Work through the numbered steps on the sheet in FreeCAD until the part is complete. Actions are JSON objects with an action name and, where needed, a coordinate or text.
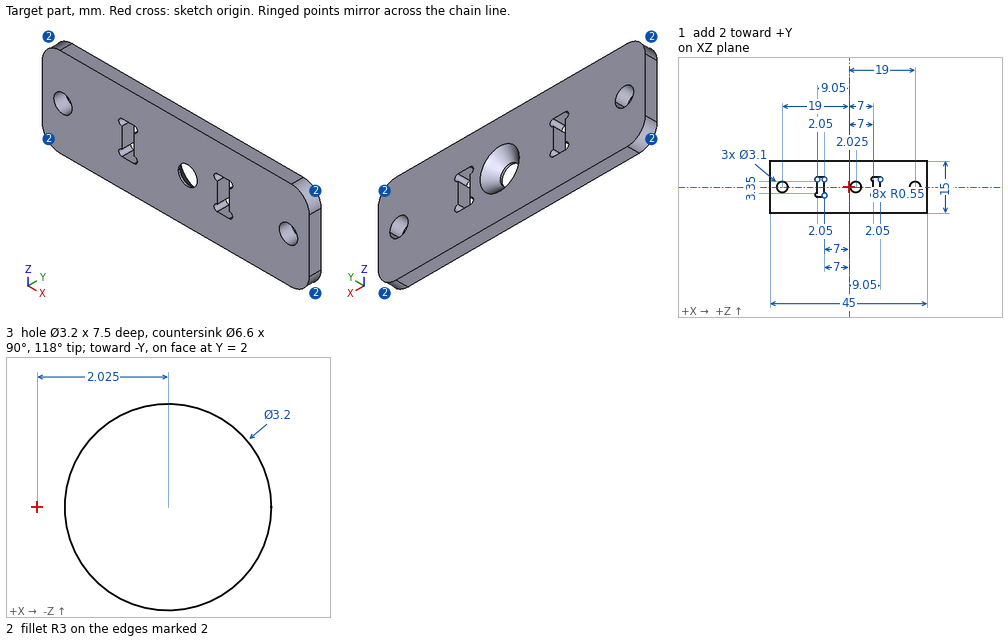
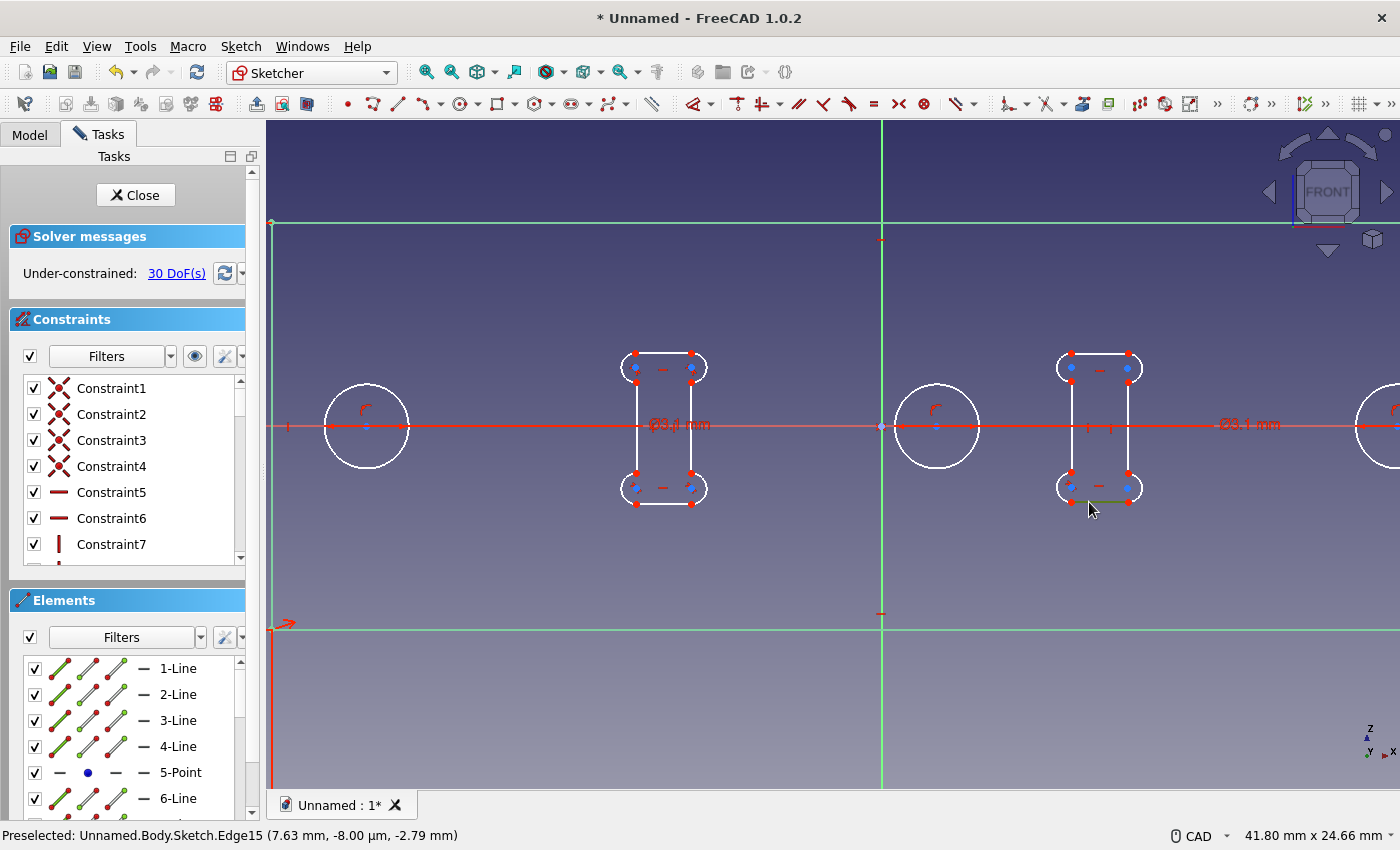
{"action": "left_click", "coordinate": [1139, 496]}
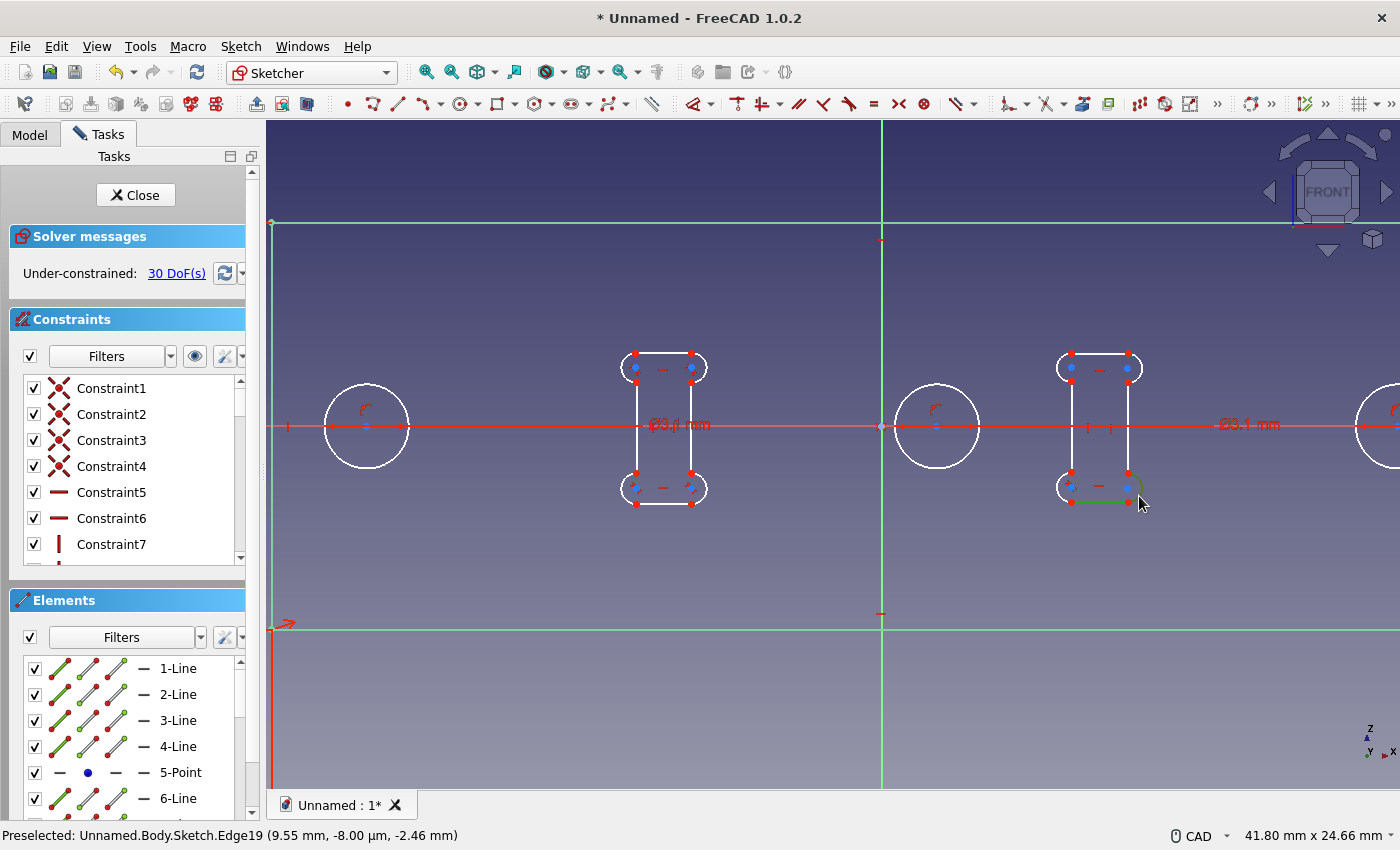
{"action": "left_click", "coordinate": [849, 104]}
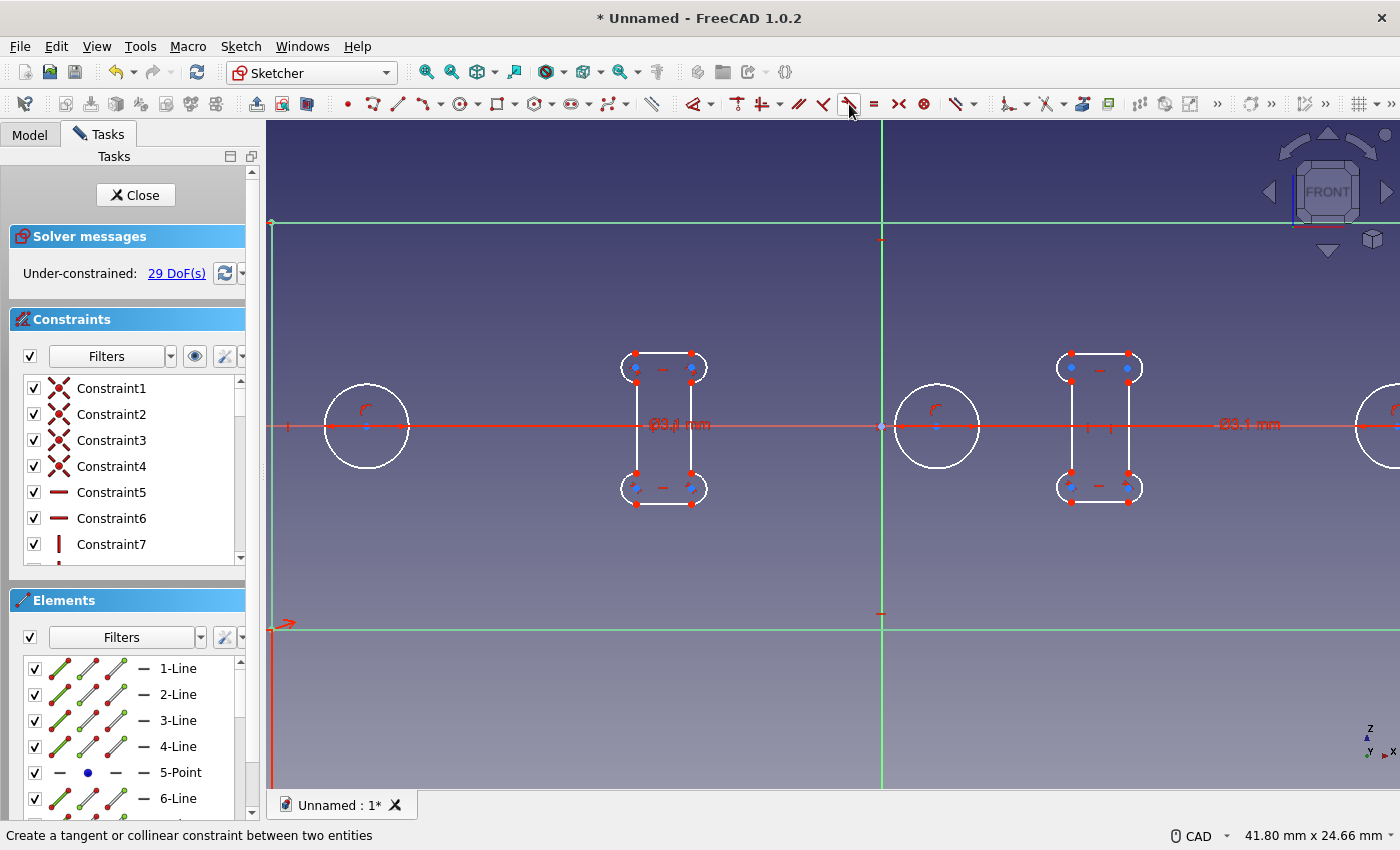
{"action": "left_click", "coordinate": [1112, 354]}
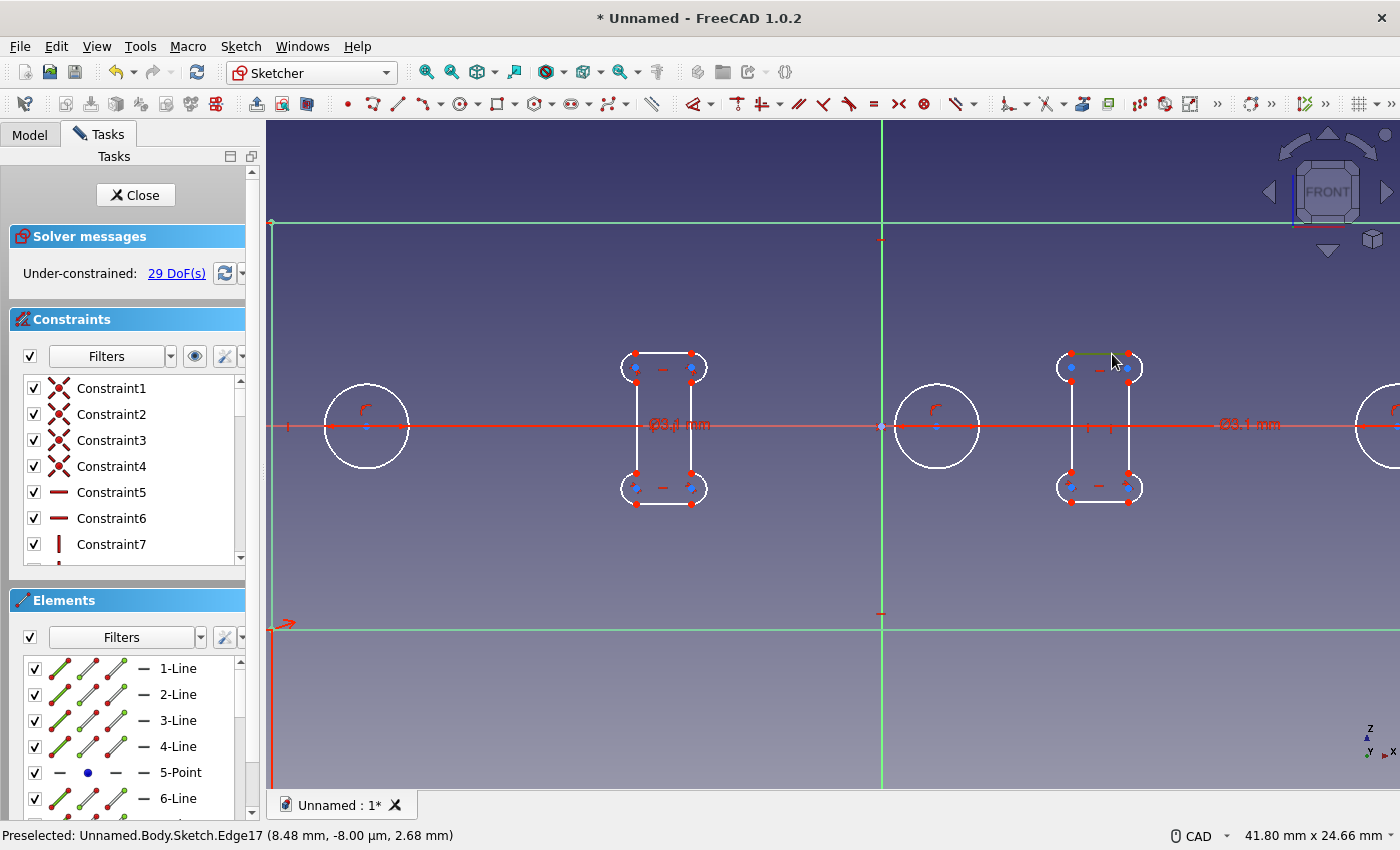
{"action": "left_click", "coordinate": [1140, 377]}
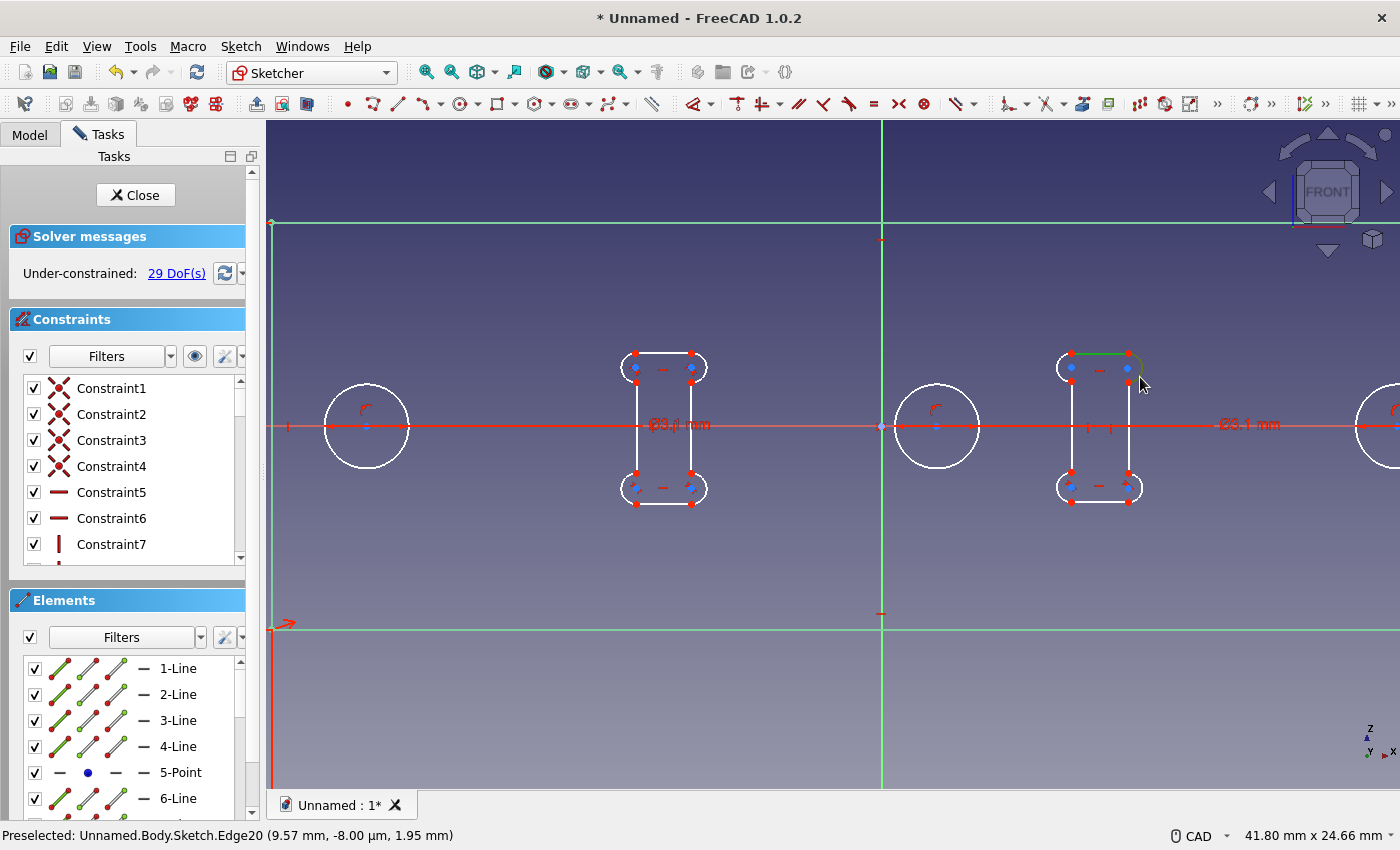
{"action": "left_click", "coordinate": [849, 104]}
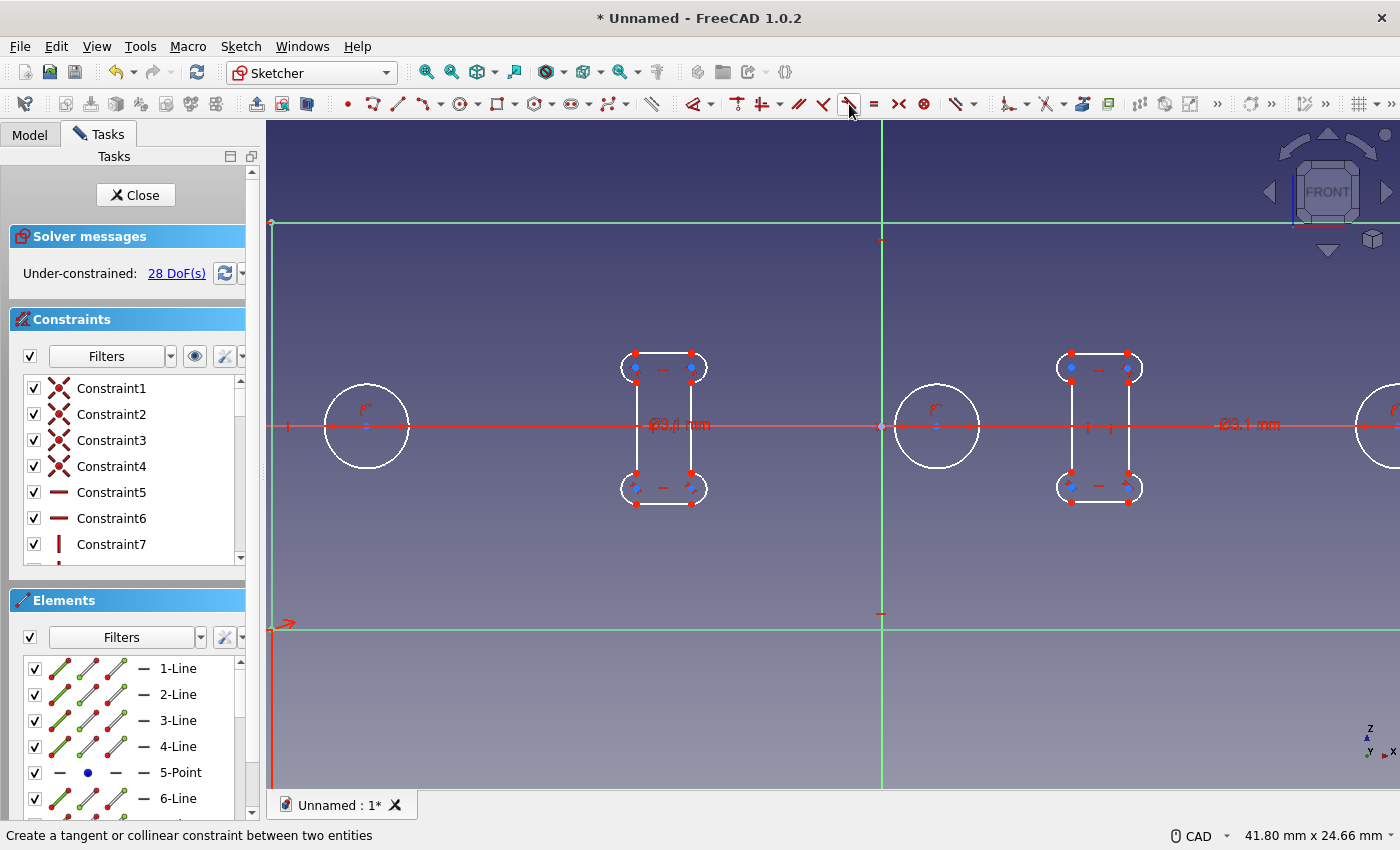
{"action": "left_click", "coordinate": [1111, 354]}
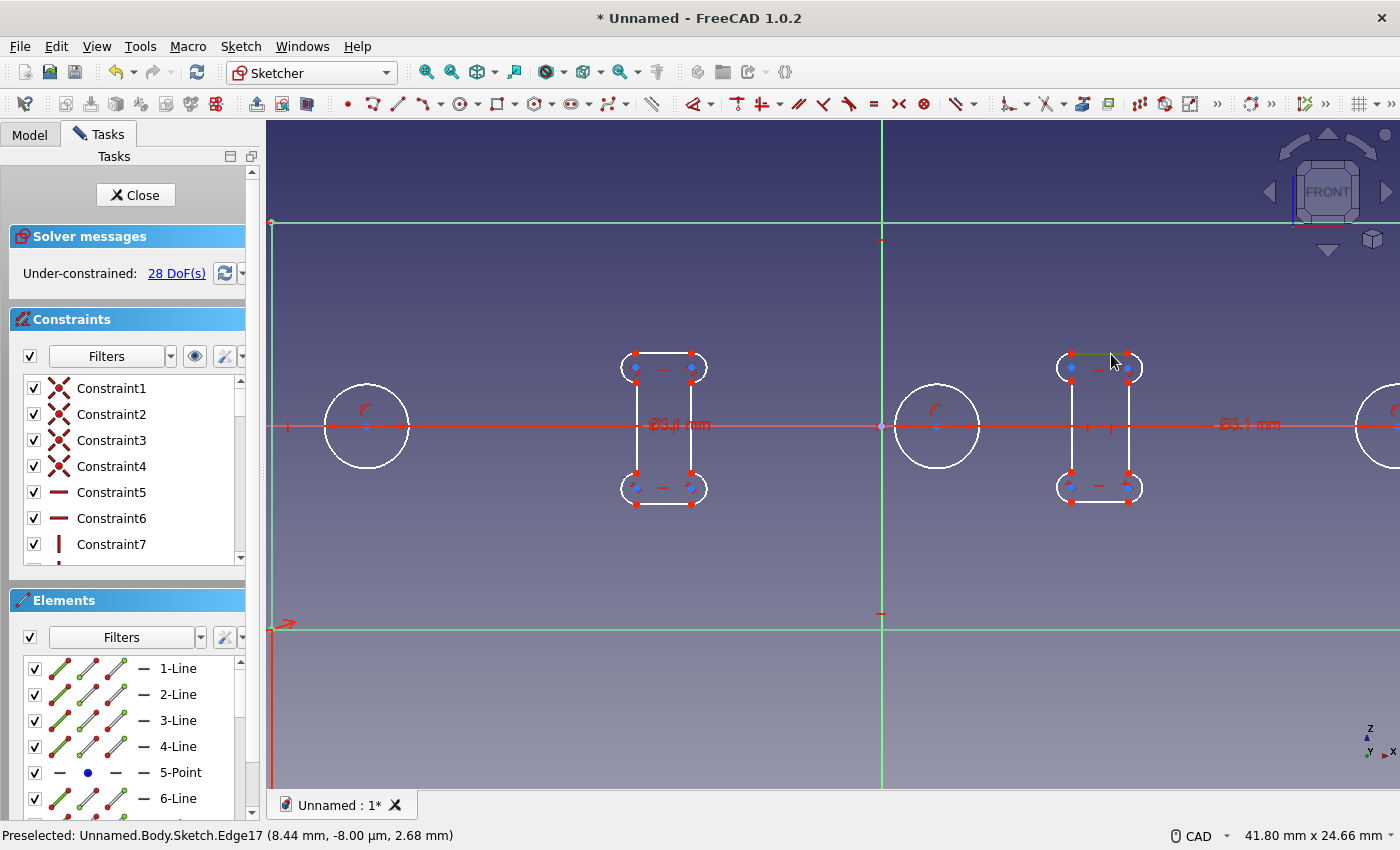
{"action": "left_click", "coordinate": [1060, 359]}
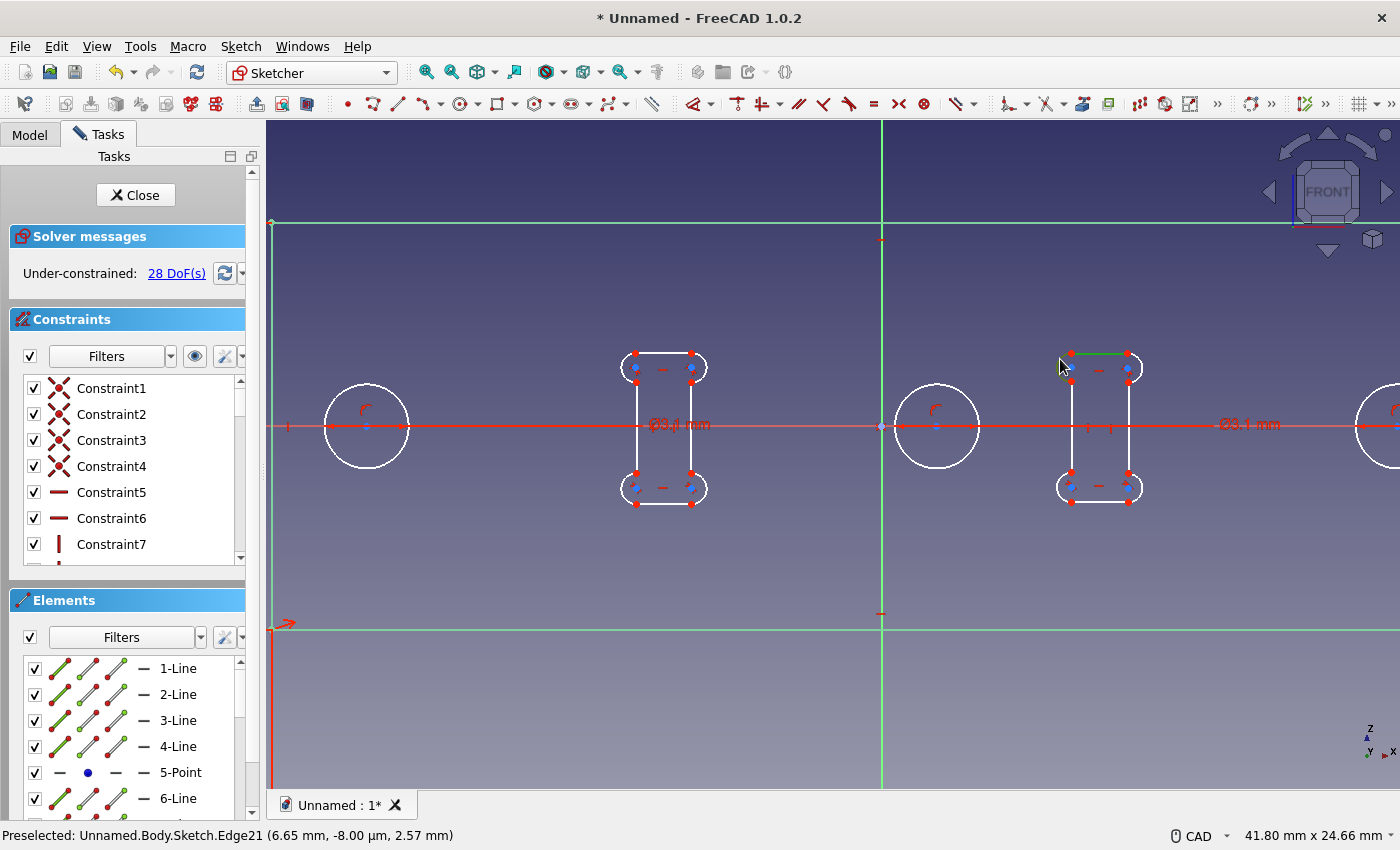
{"action": "left_click", "coordinate": [849, 104]}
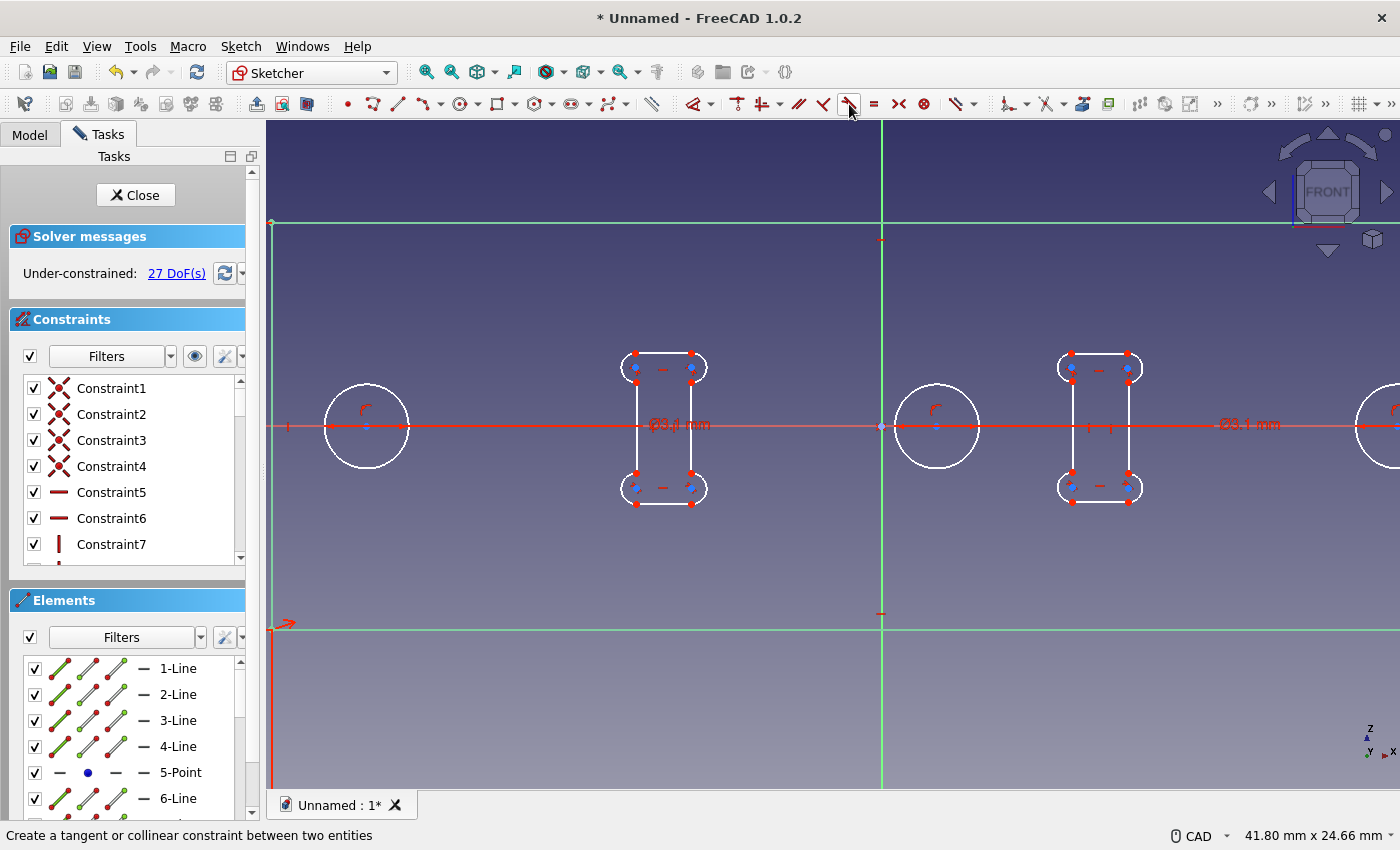
{"action": "left_click", "coordinate": [624, 480]}